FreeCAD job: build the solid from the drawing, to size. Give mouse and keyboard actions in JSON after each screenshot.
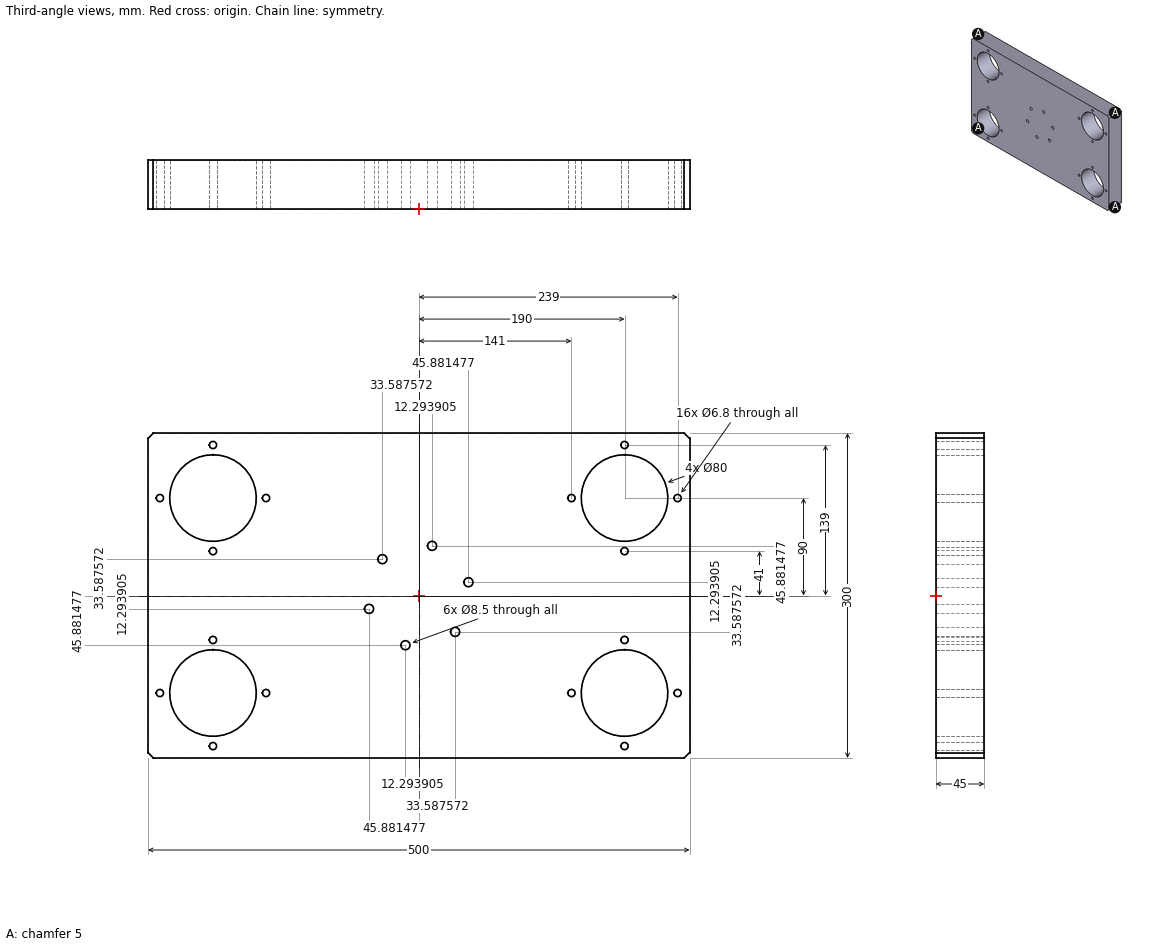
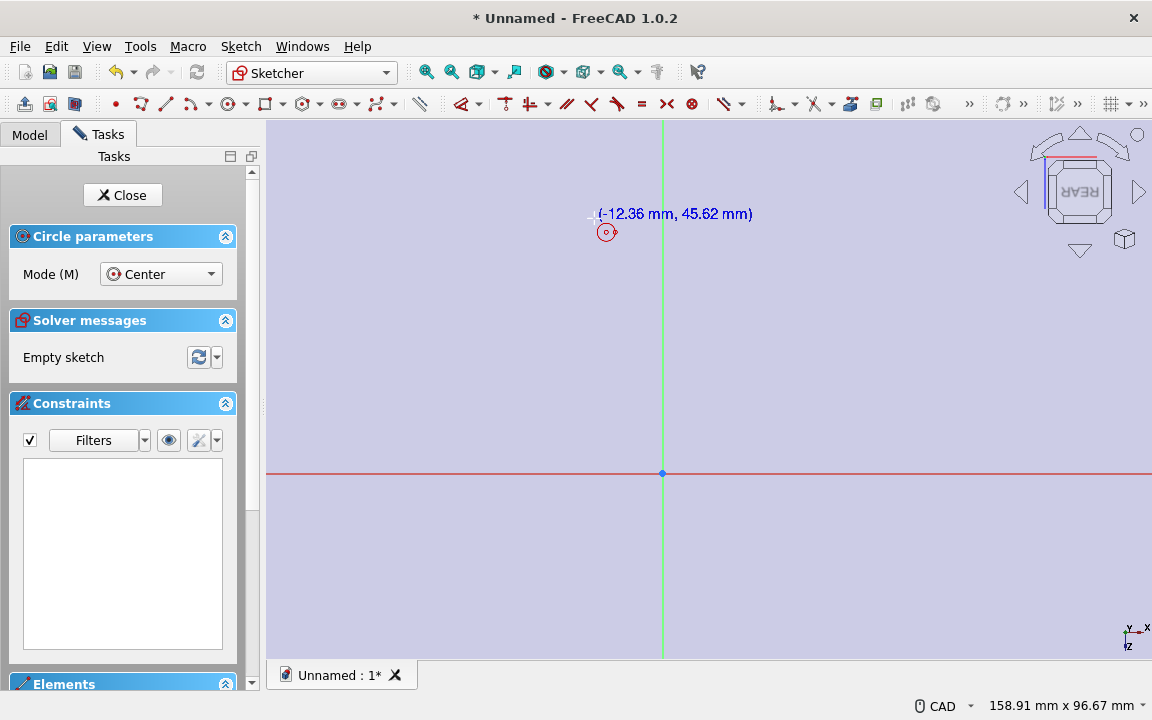
{"action": "left_click", "coordinate": [594, 218]}
{"action": "left_click", "coordinate": [611, 201]}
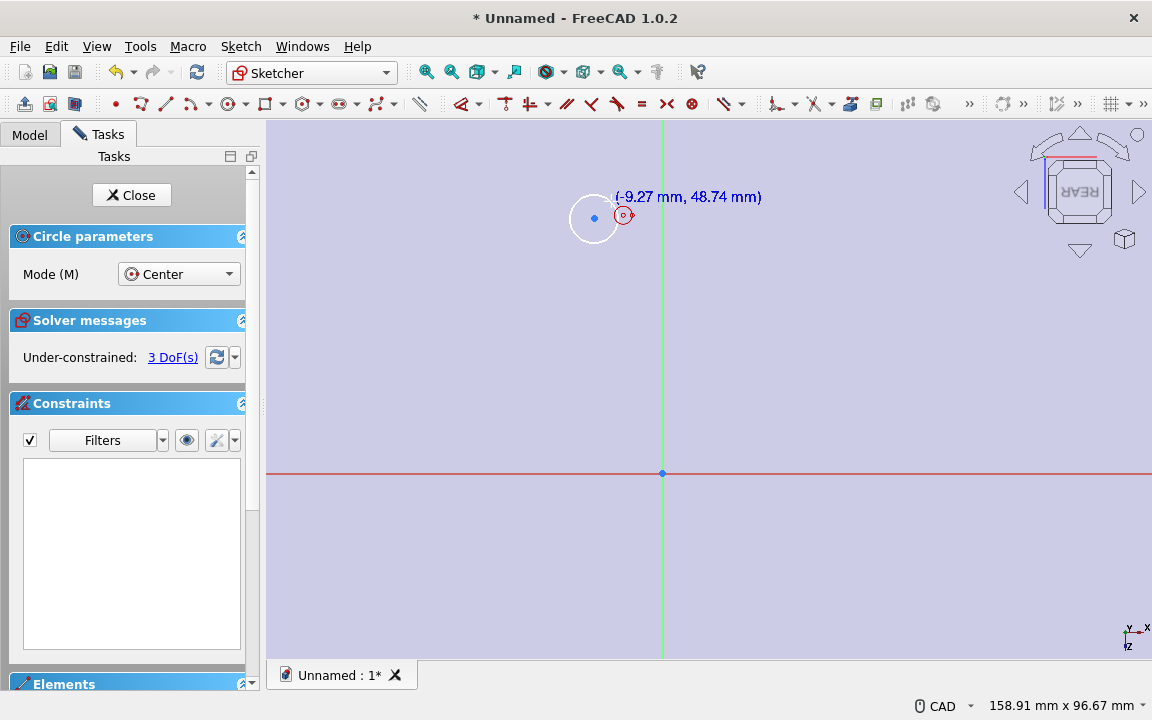
{"action": "left_click", "coordinate": [407, 405]}
{"action": "left_click", "coordinate": [424, 388]}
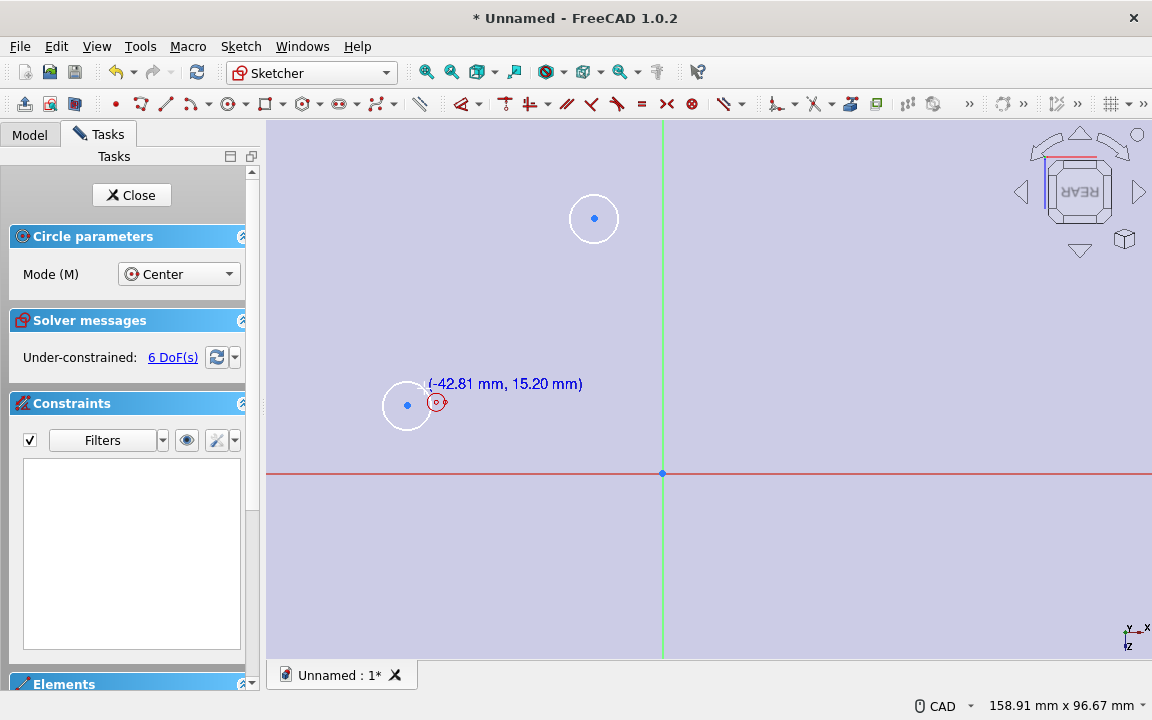
{"action": "scroll", "coordinate": [595, 218], "scroll_direction": "down", "scroll_amount": 2}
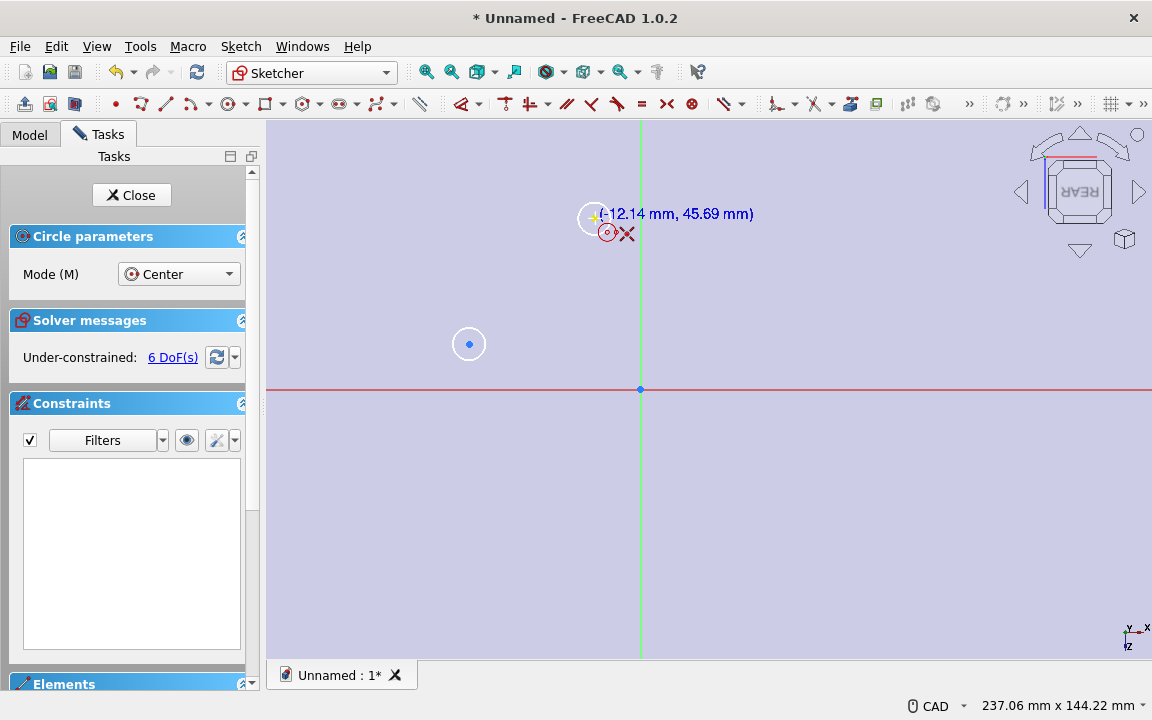
{"action": "scroll", "coordinate": [515, 515], "scroll_direction": "up", "scroll_amount": 2}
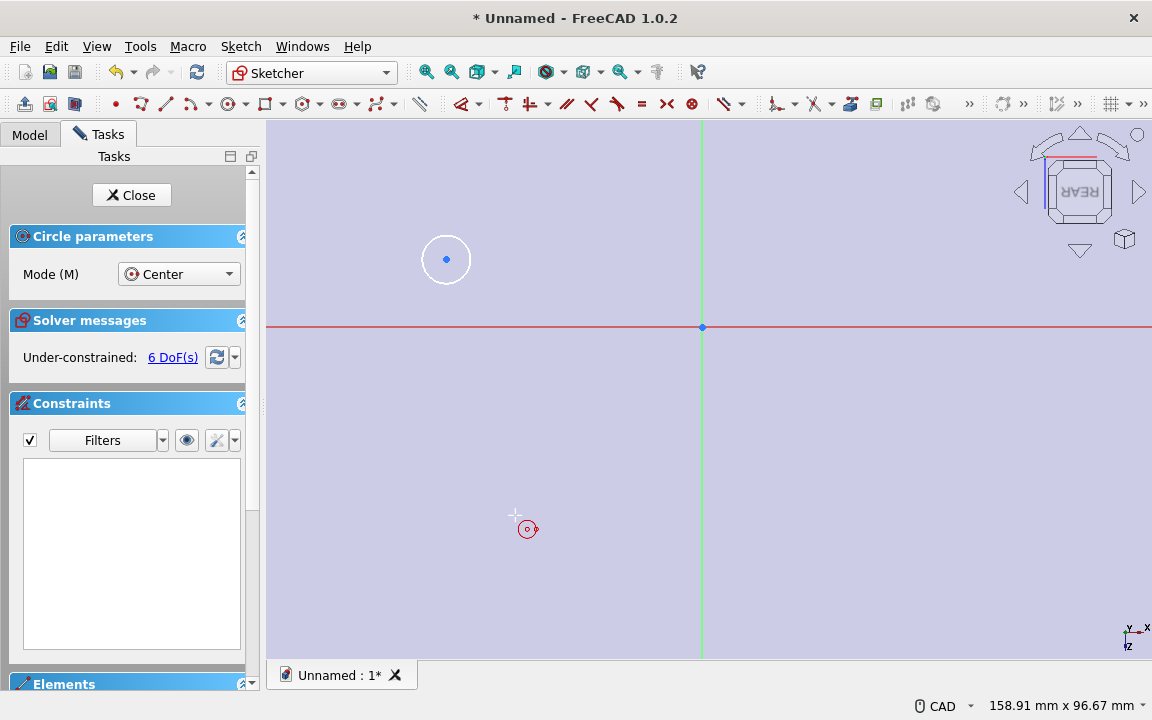
{"action": "left_click", "coordinate": [515, 515]}
{"action": "left_click", "coordinate": [532, 498]}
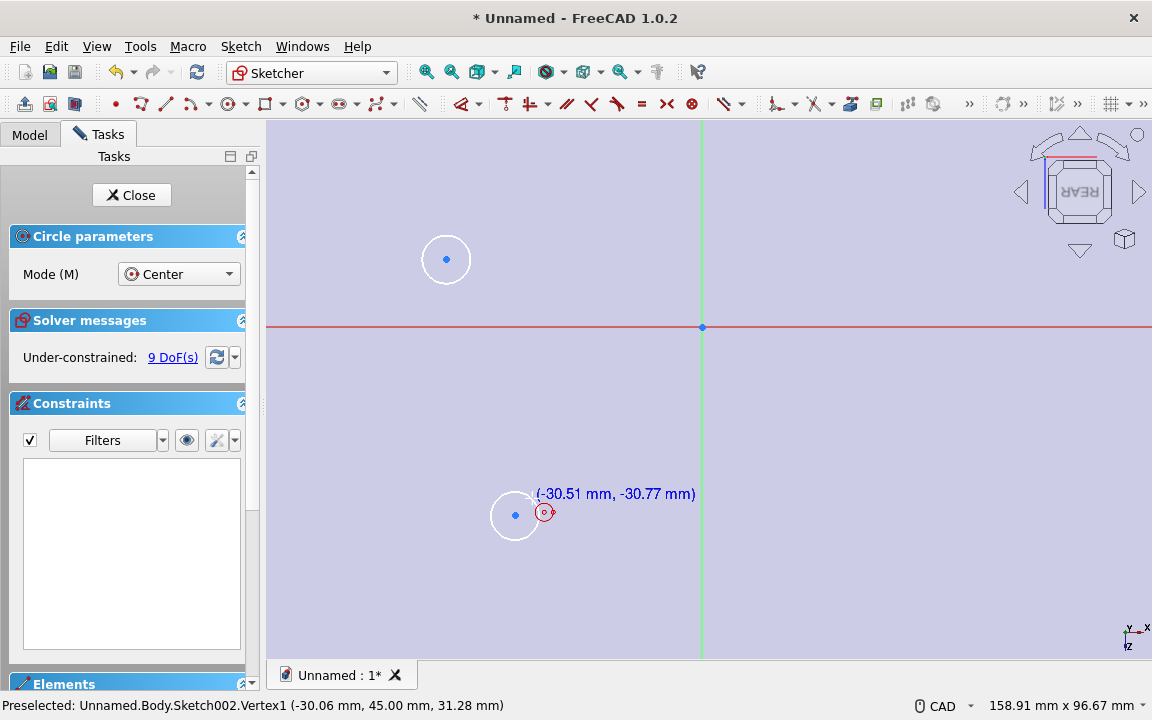
{"action": "left_click", "coordinate": [771, 583]}
{"action": "left_click", "coordinate": [787, 566]}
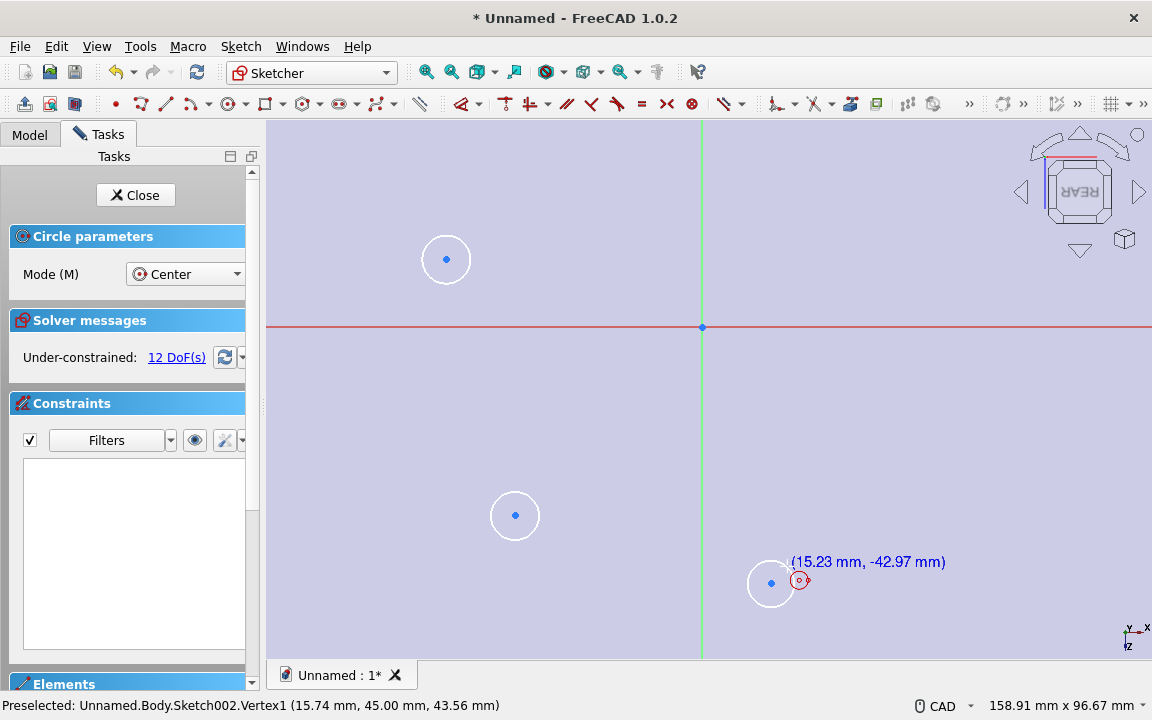
{"action": "left_click", "coordinate": [958, 396]}
{"action": "left_click", "coordinate": [975, 379]}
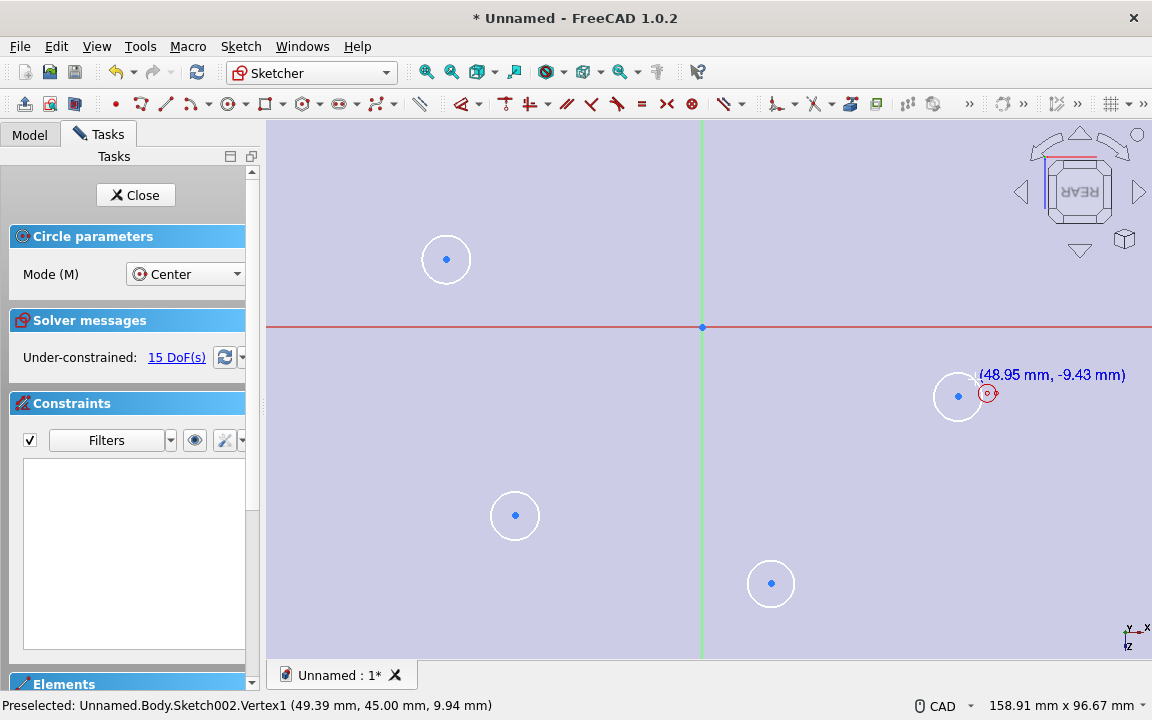
{"action": "scroll", "coordinate": [515, 516], "scroll_direction": "down", "scroll_amount": 2}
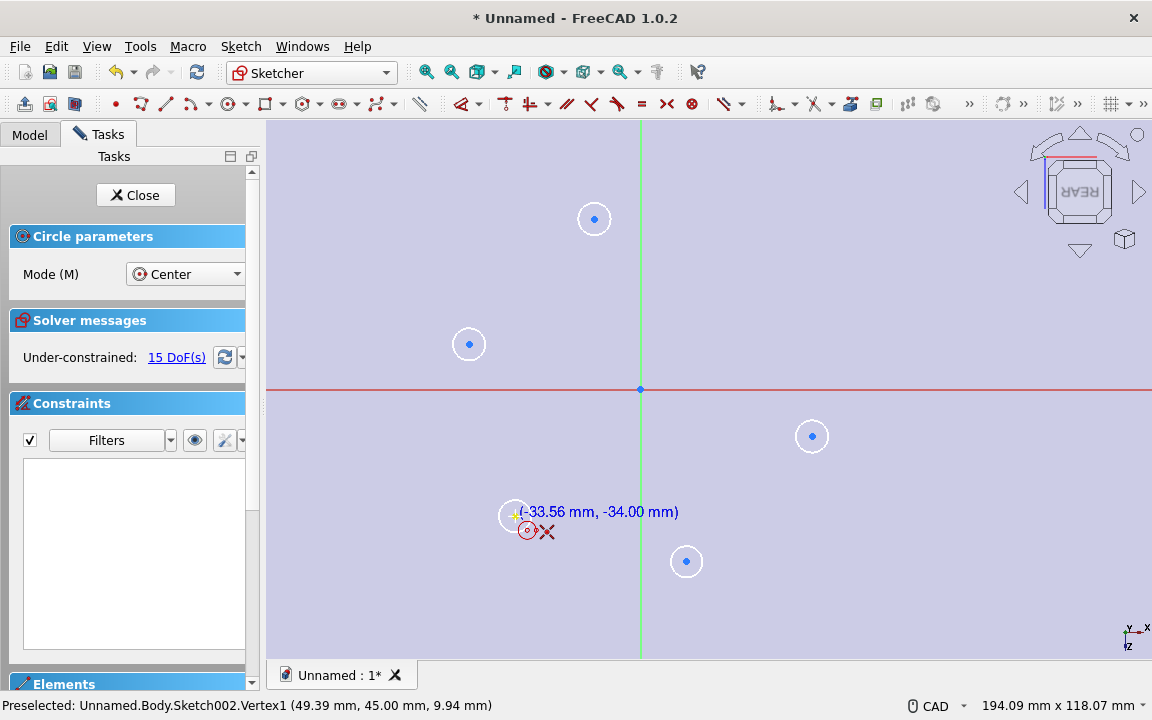
{"action": "scroll", "coordinate": [766, 264], "scroll_direction": "up", "scroll_amount": 2}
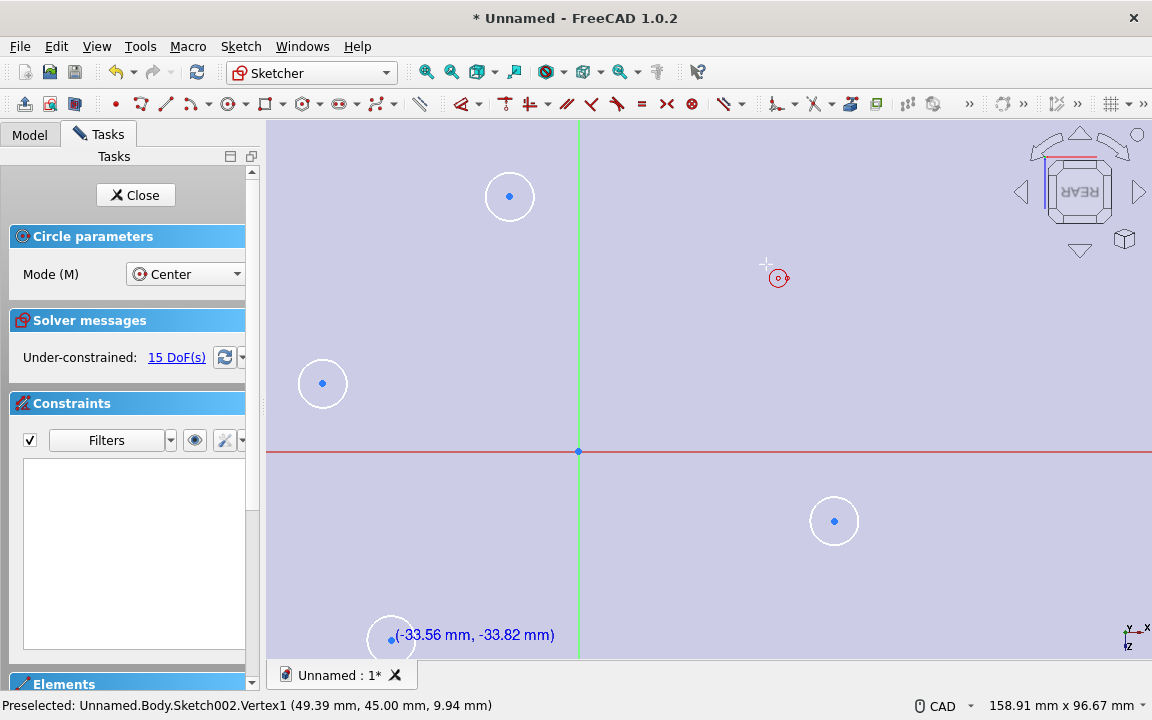
{"action": "left_click", "coordinate": [766, 264]}
{"action": "left_click", "coordinate": [783, 248]}
{"action": "key", "text": "Escape"}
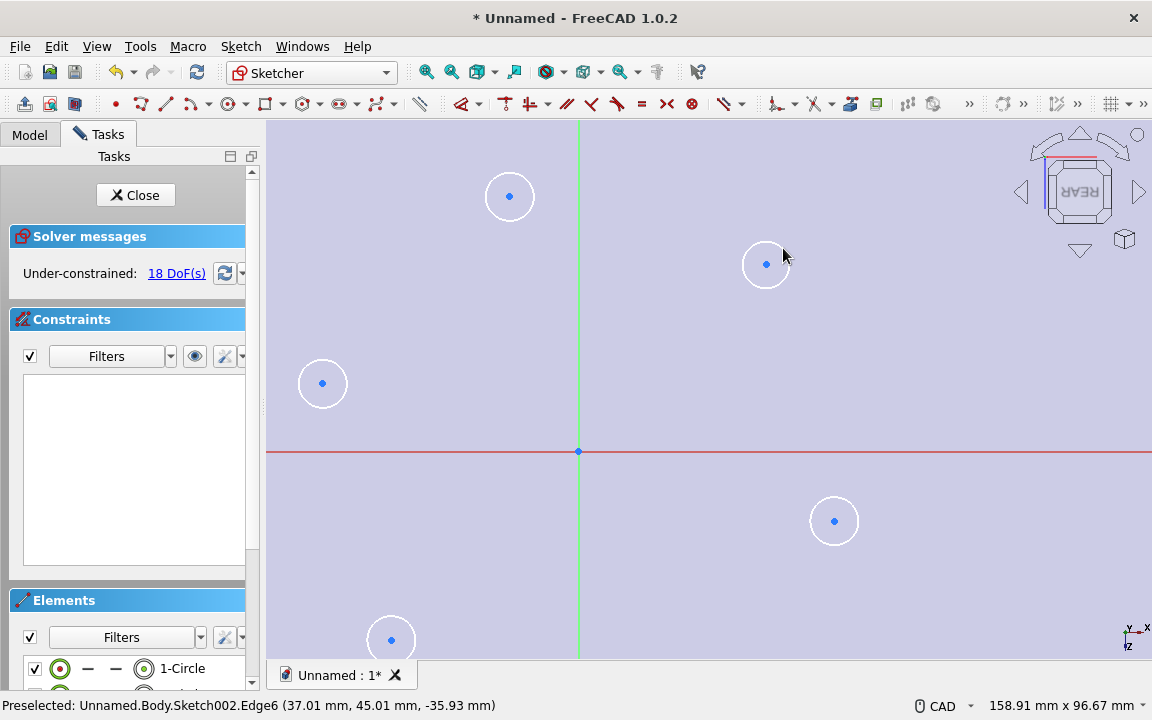
{"action": "left_click", "coordinate": [527, 180]}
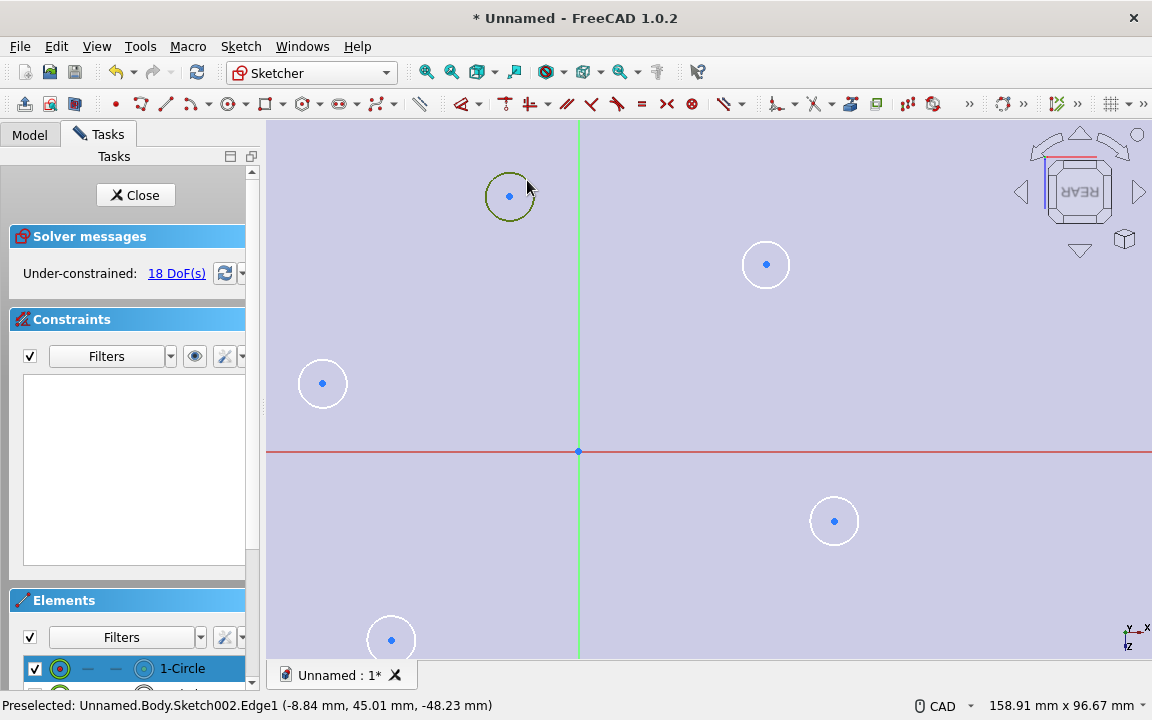
{"action": "left_click", "coordinate": [340, 367]}